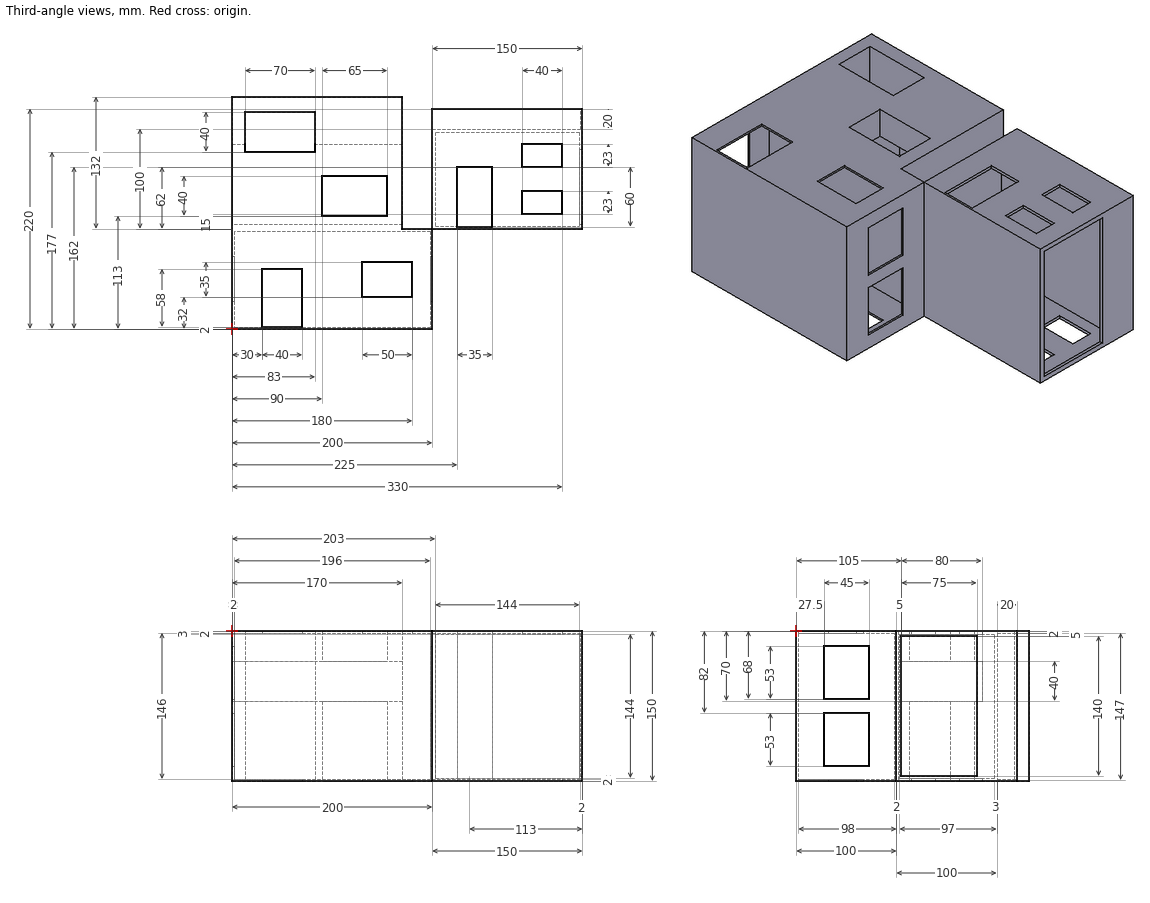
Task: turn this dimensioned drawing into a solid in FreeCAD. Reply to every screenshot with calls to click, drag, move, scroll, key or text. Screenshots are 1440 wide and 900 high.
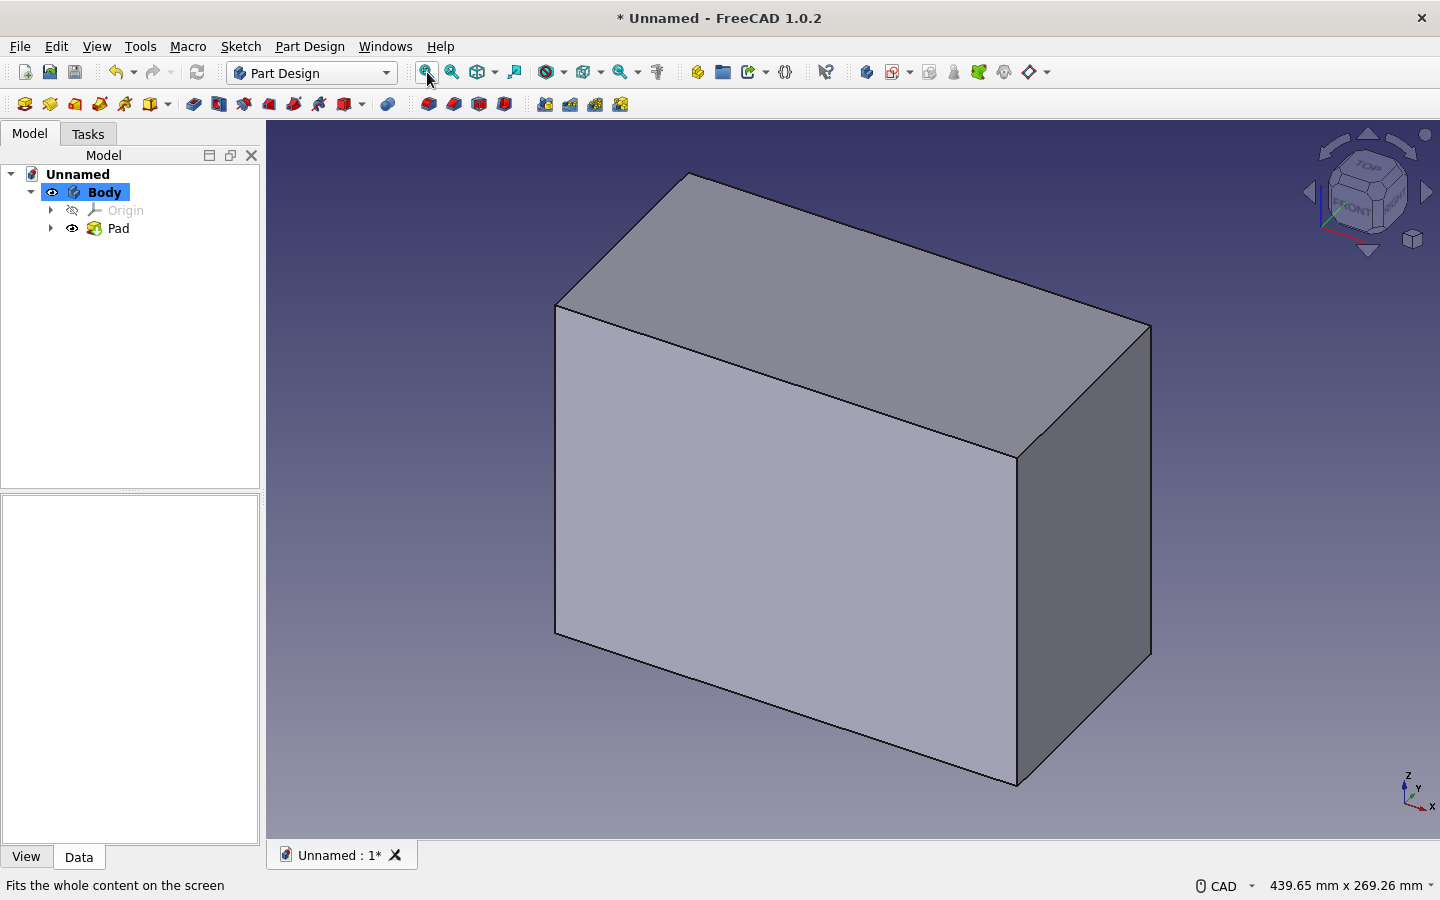
click(892, 72)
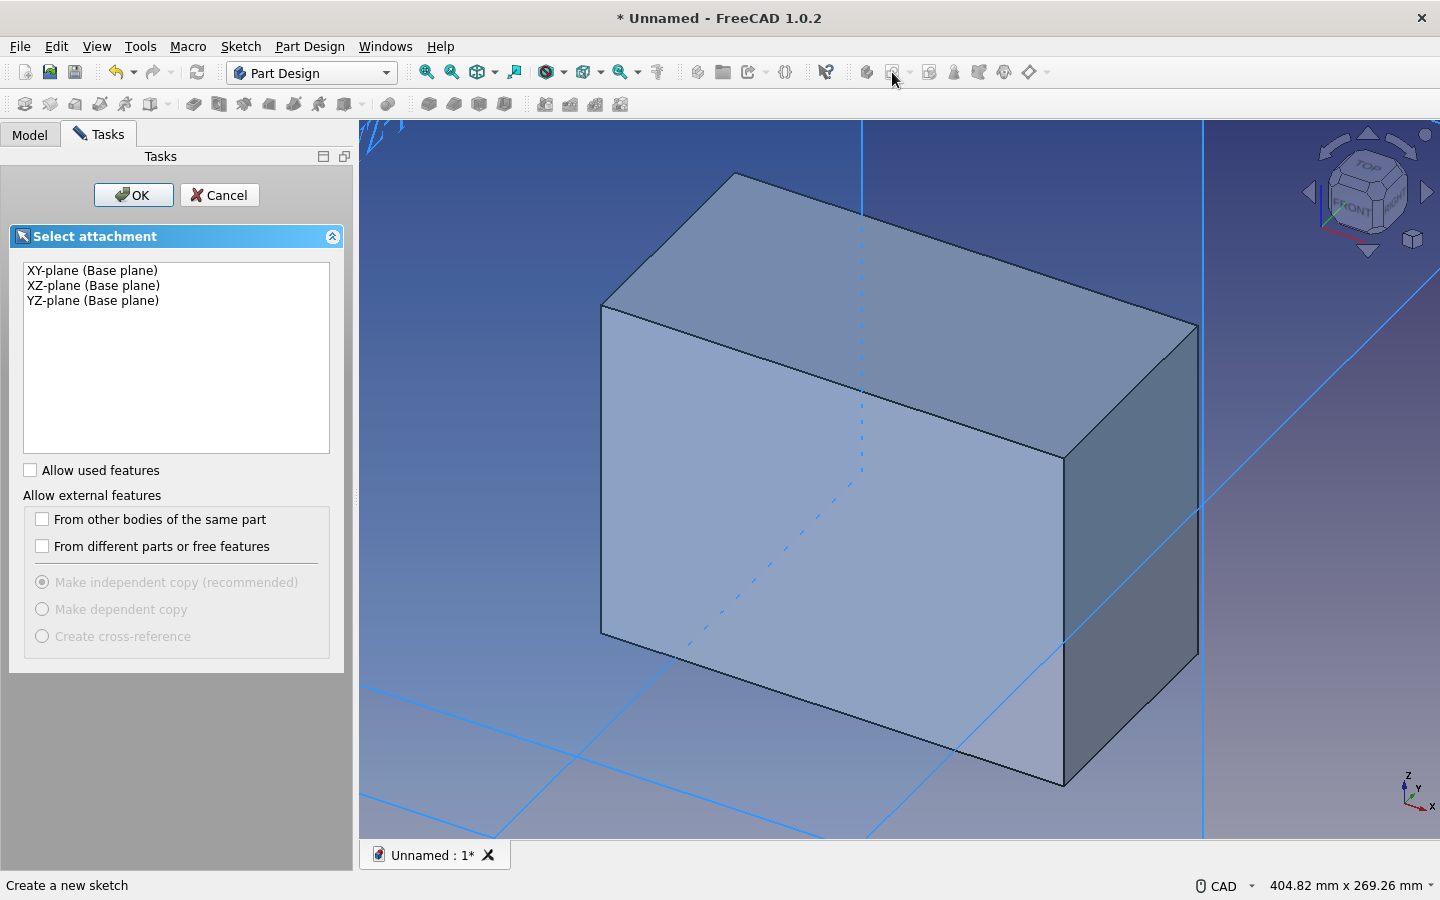
click(84, 270)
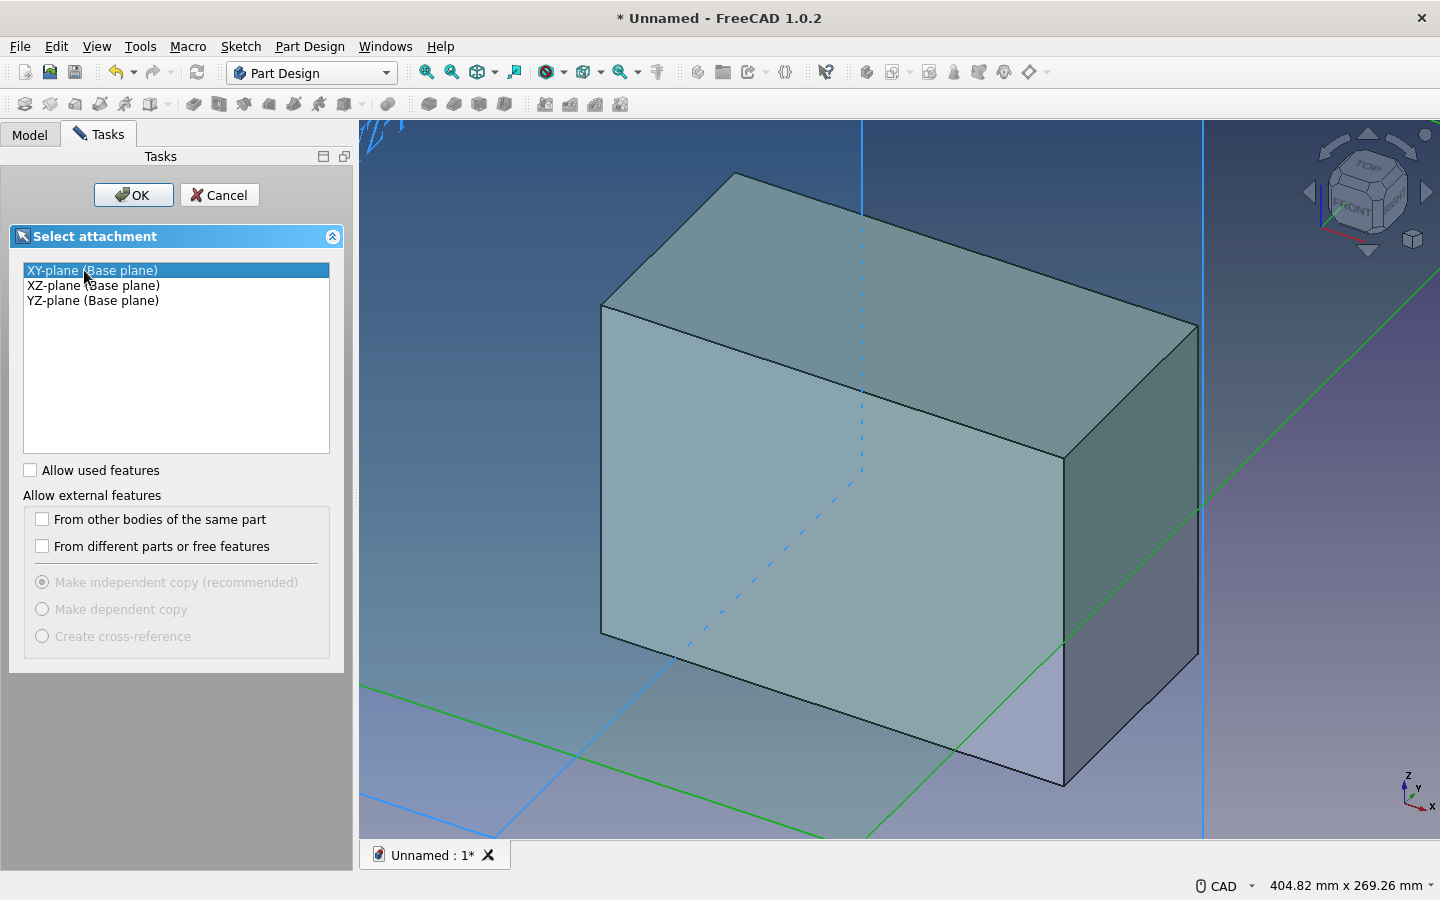
click(134, 195)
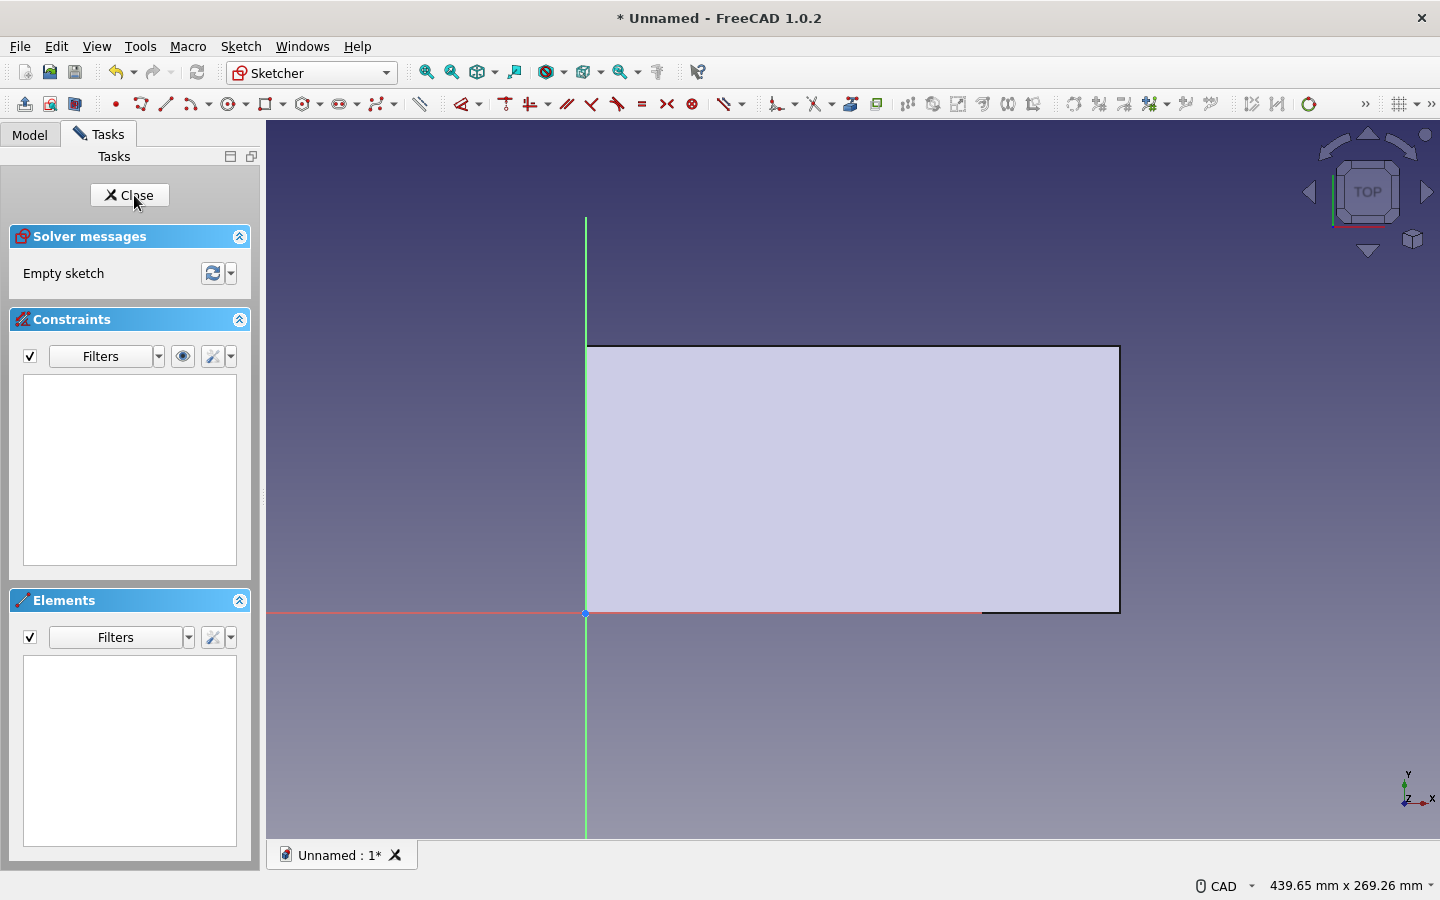
scroll(618, 564, up, 5)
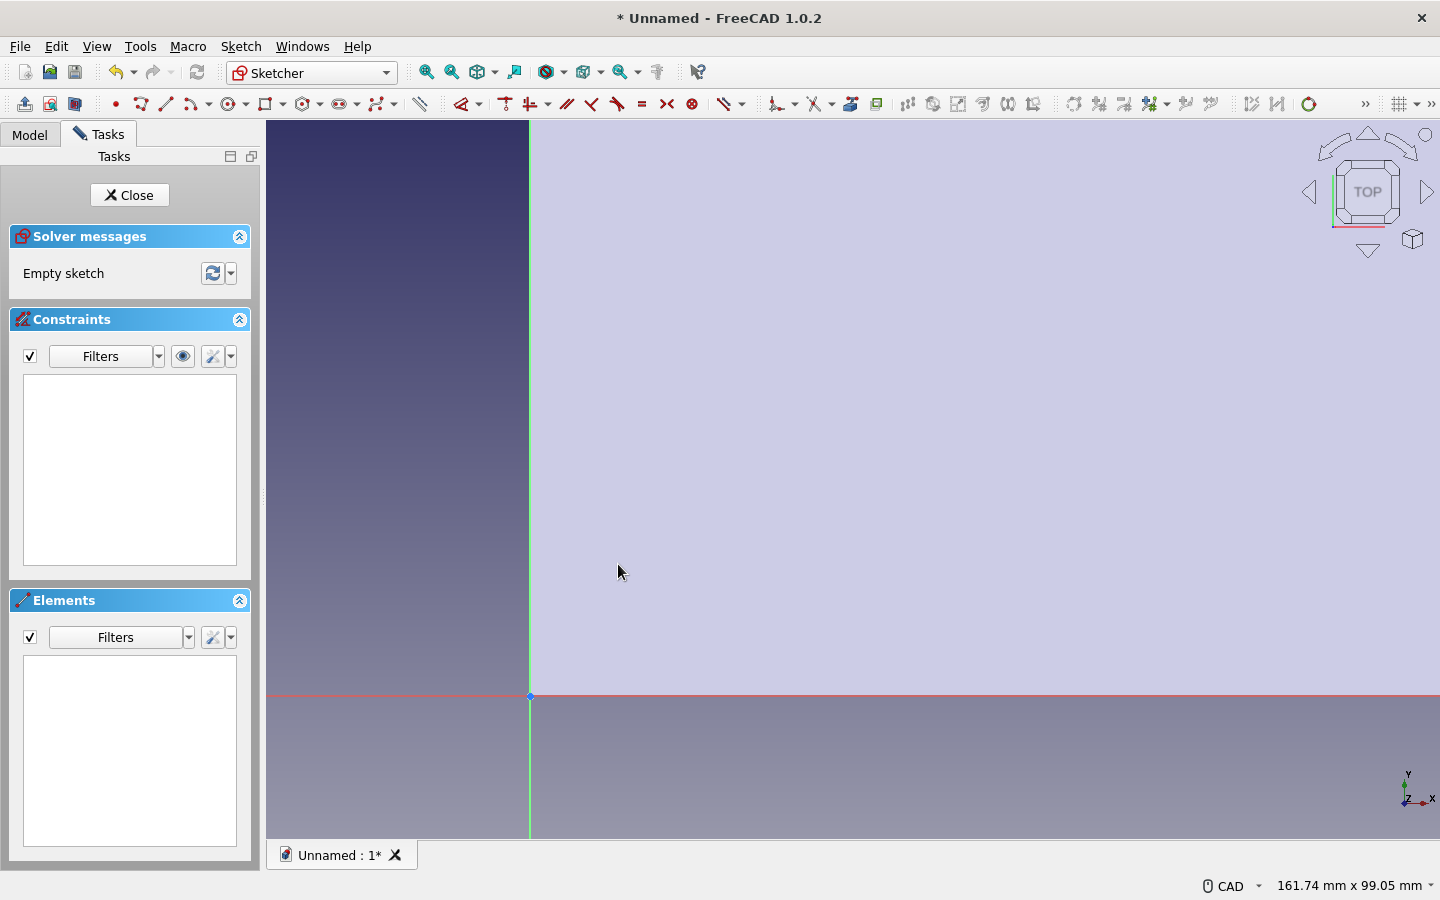
click(264, 104)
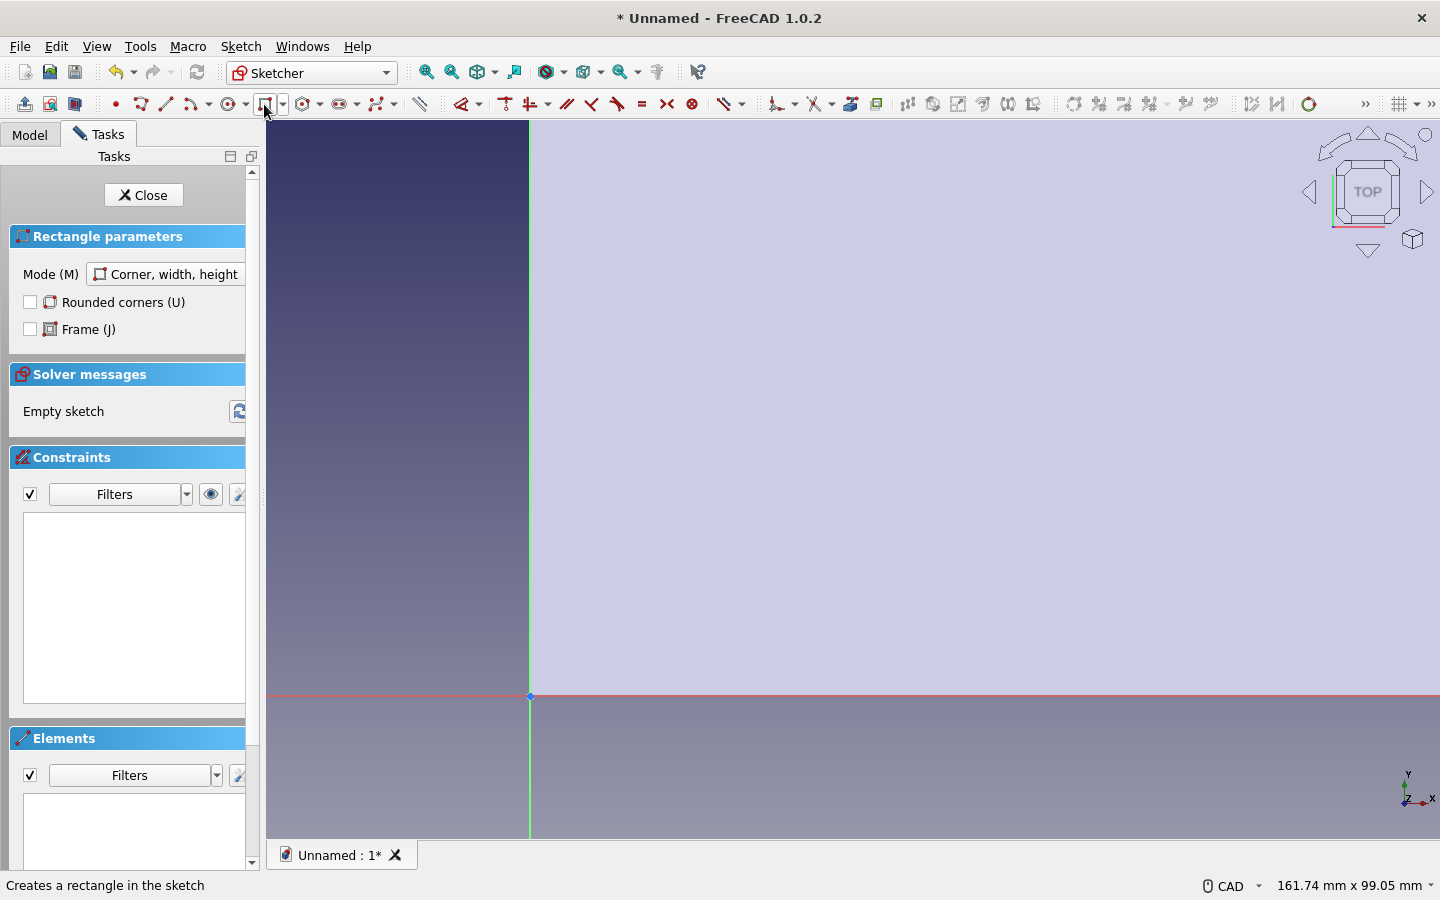
click(748, 261)
move(1039, 682)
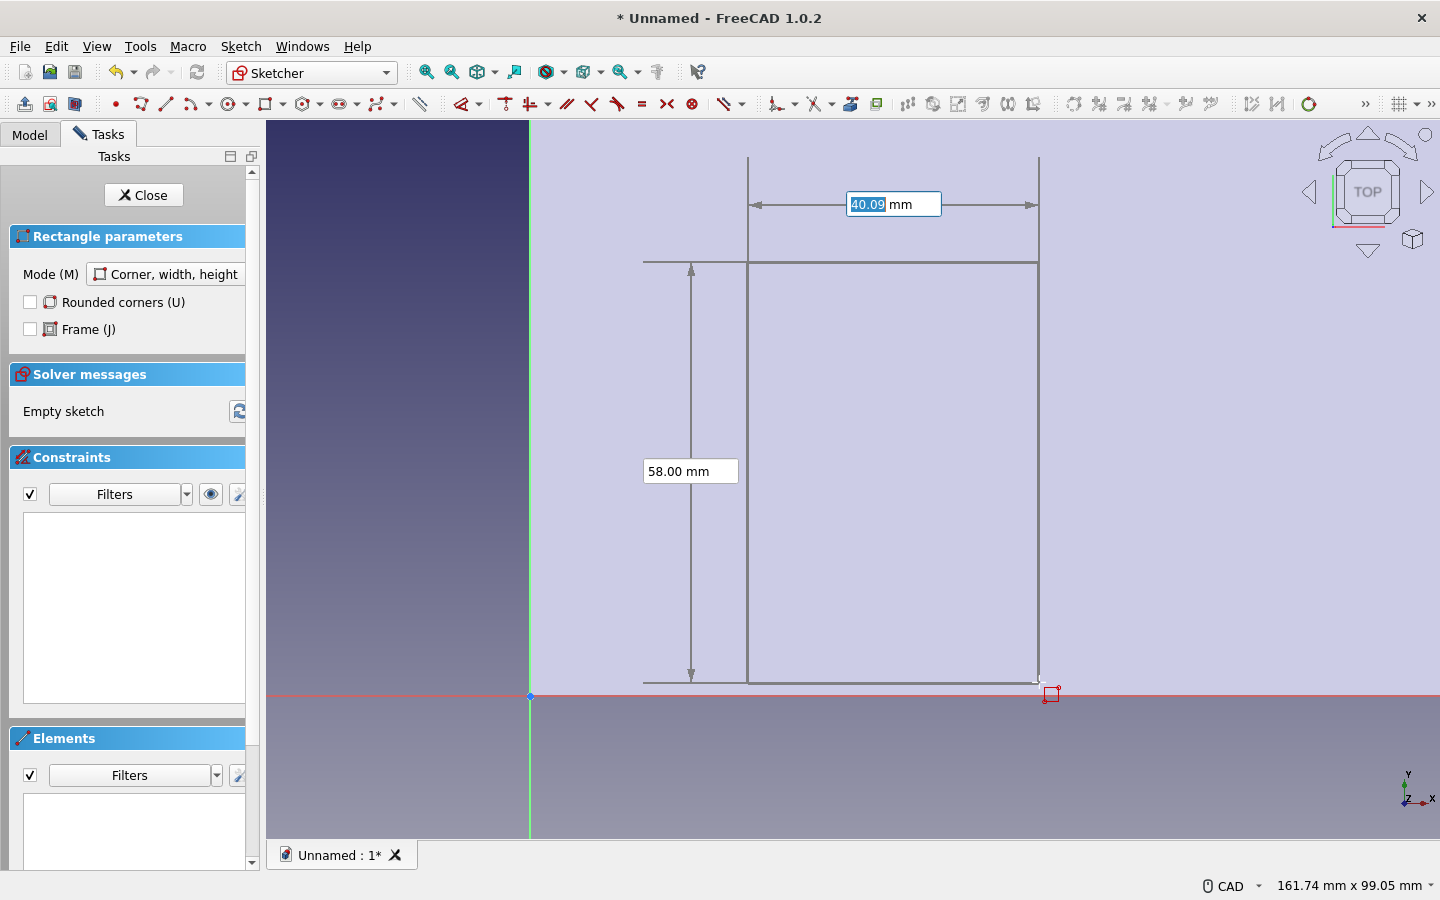
text(40)
key(Tab)
text(58)
key(Return)
key(Escape)